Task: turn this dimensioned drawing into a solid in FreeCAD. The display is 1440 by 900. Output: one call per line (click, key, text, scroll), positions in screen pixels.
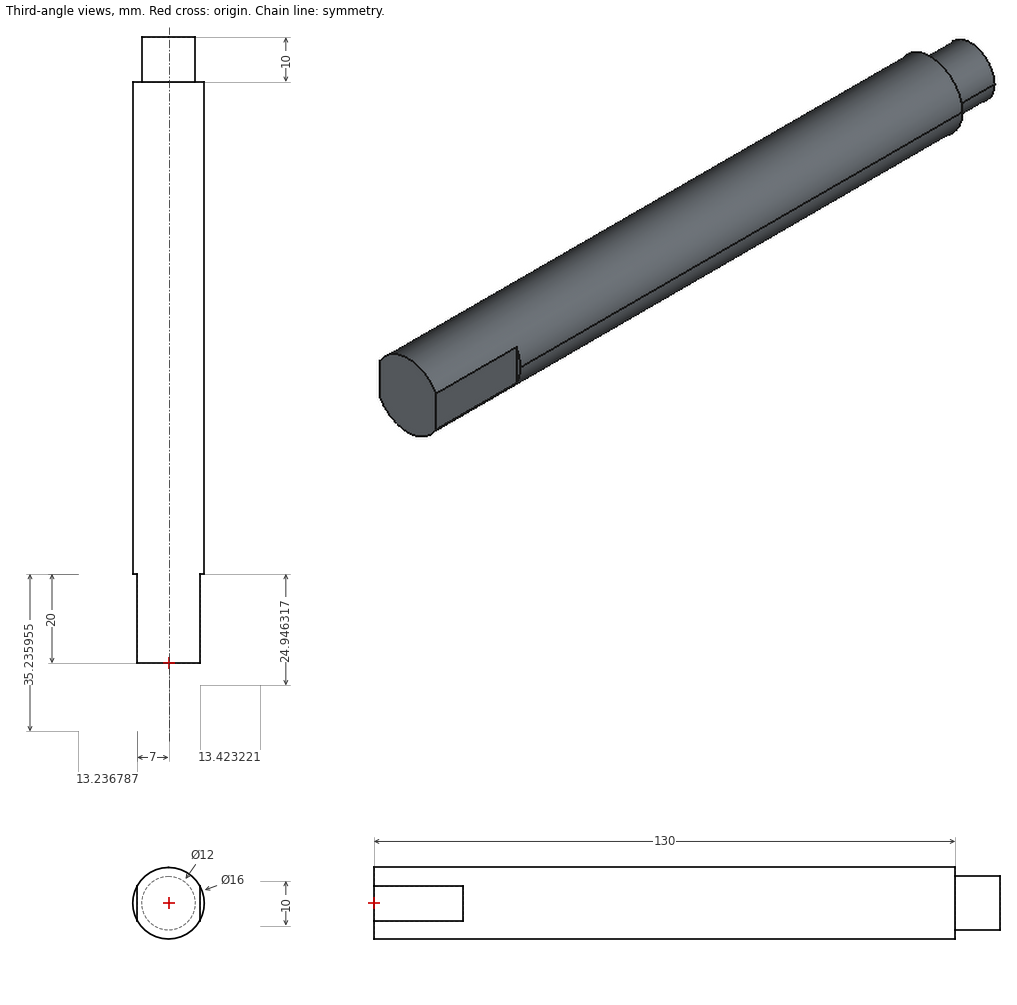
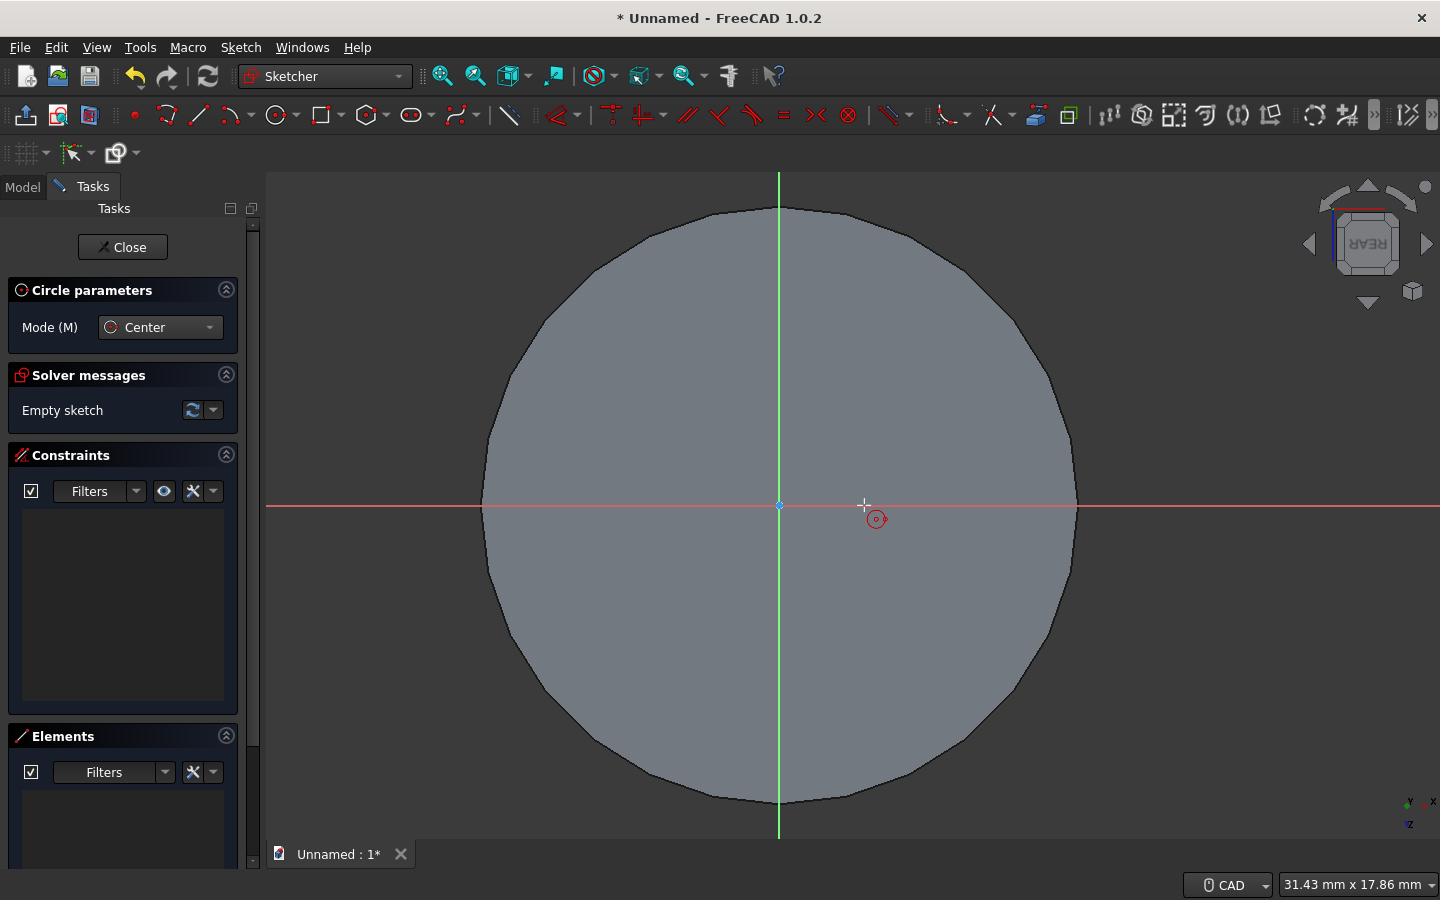
click(779, 505)
click(938, 347)
key(Escape)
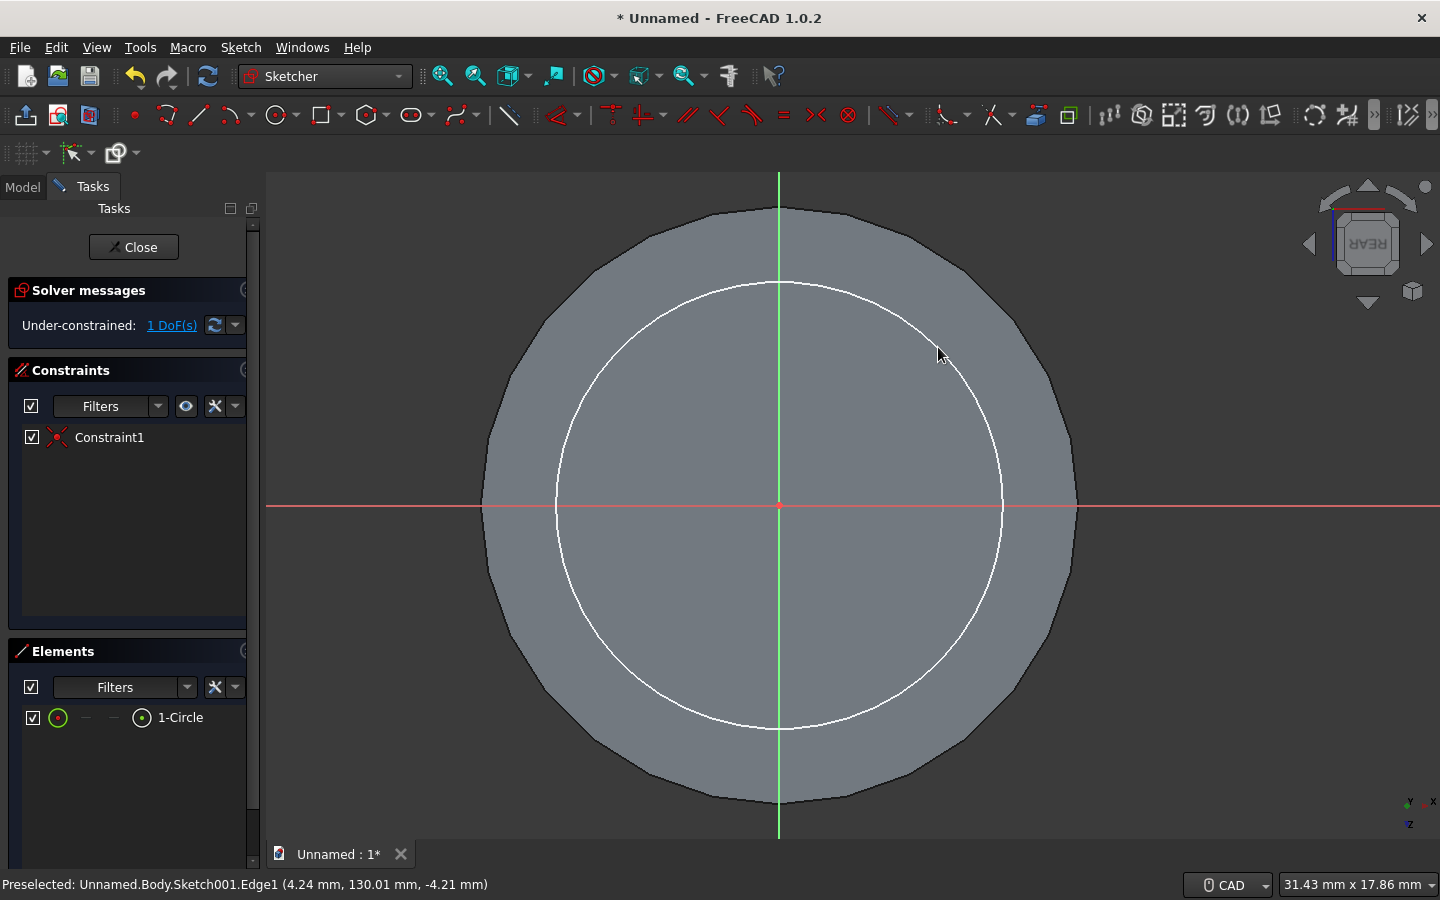
click(556, 116)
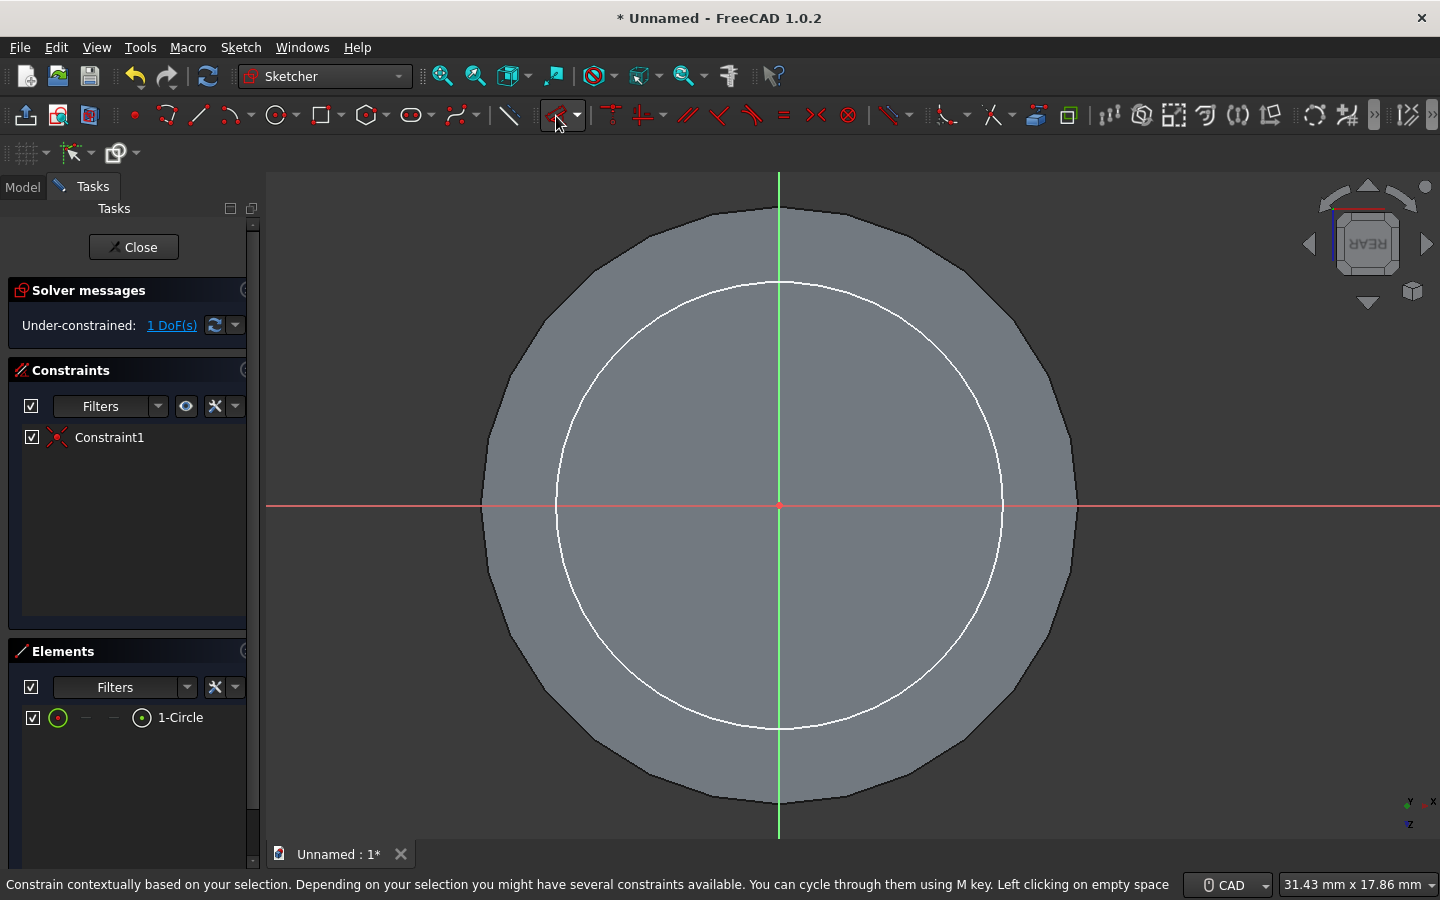
click(937, 347)
click(960, 324)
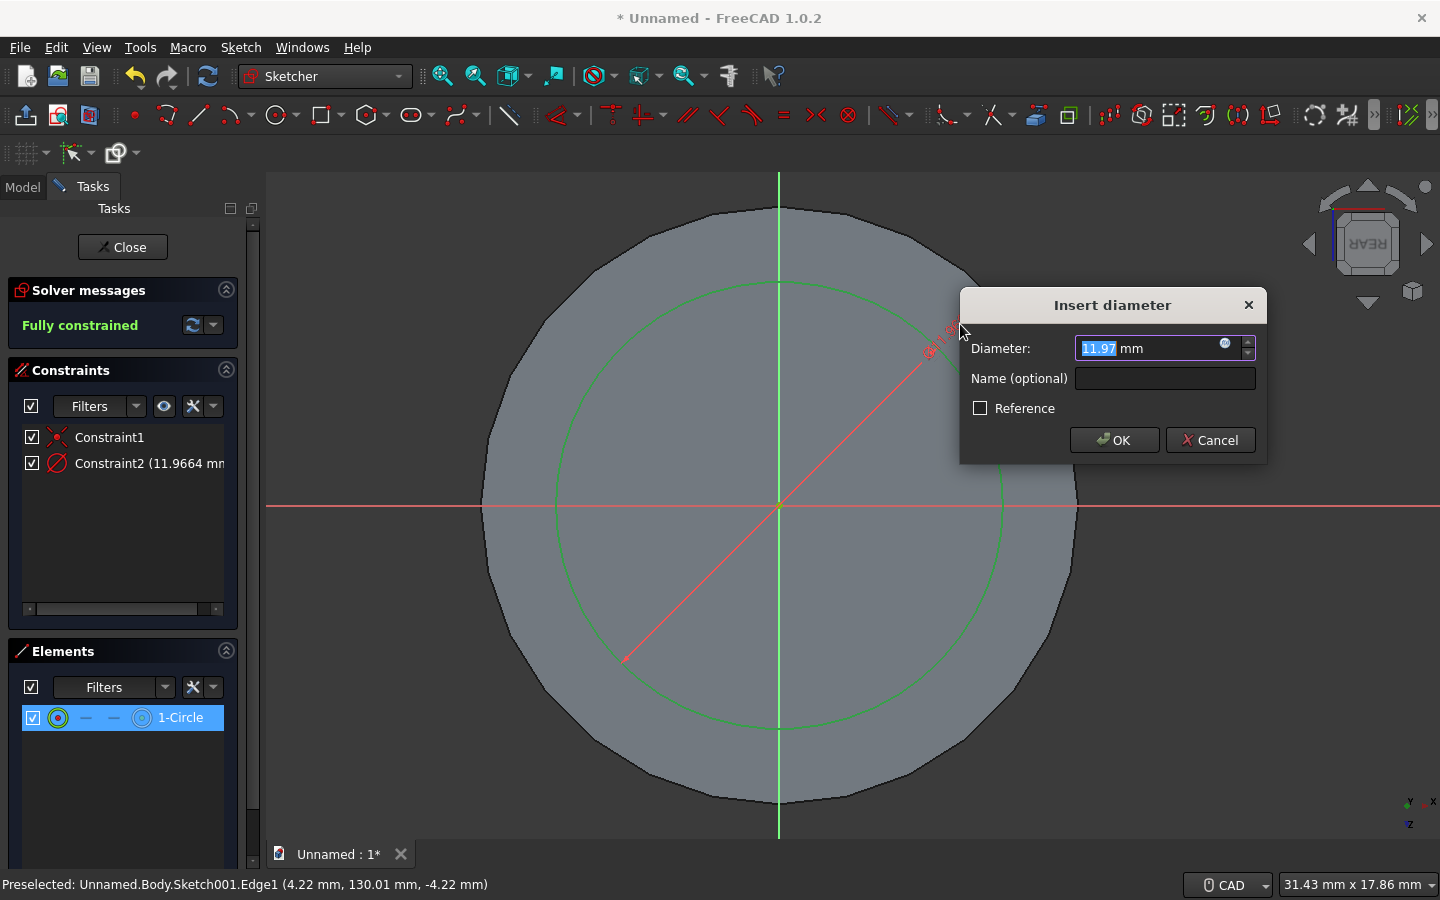
text(12)
key(Return)
key(Escape)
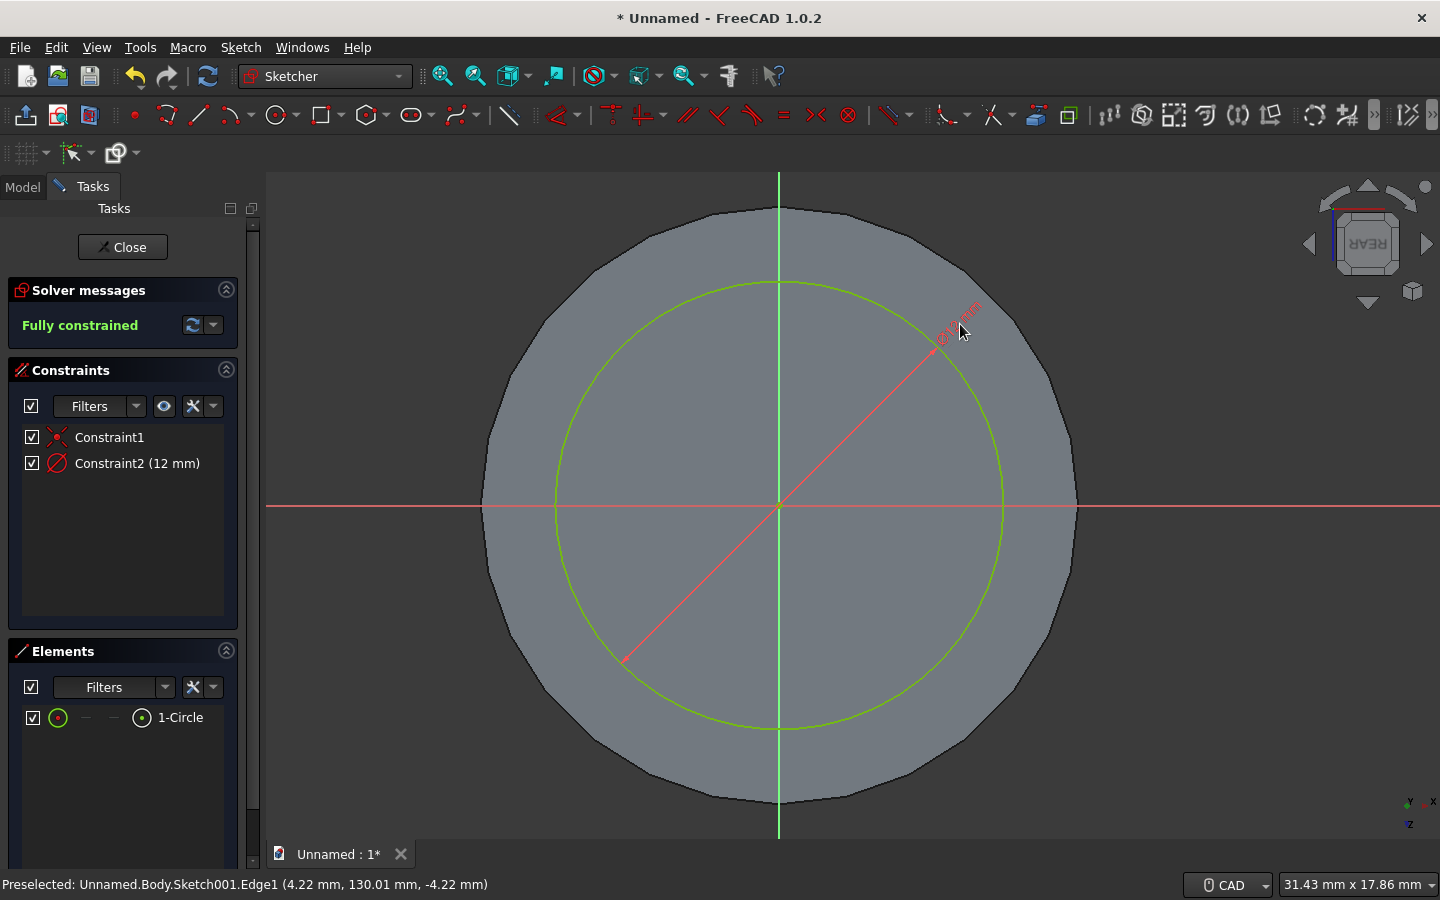
click(123, 247)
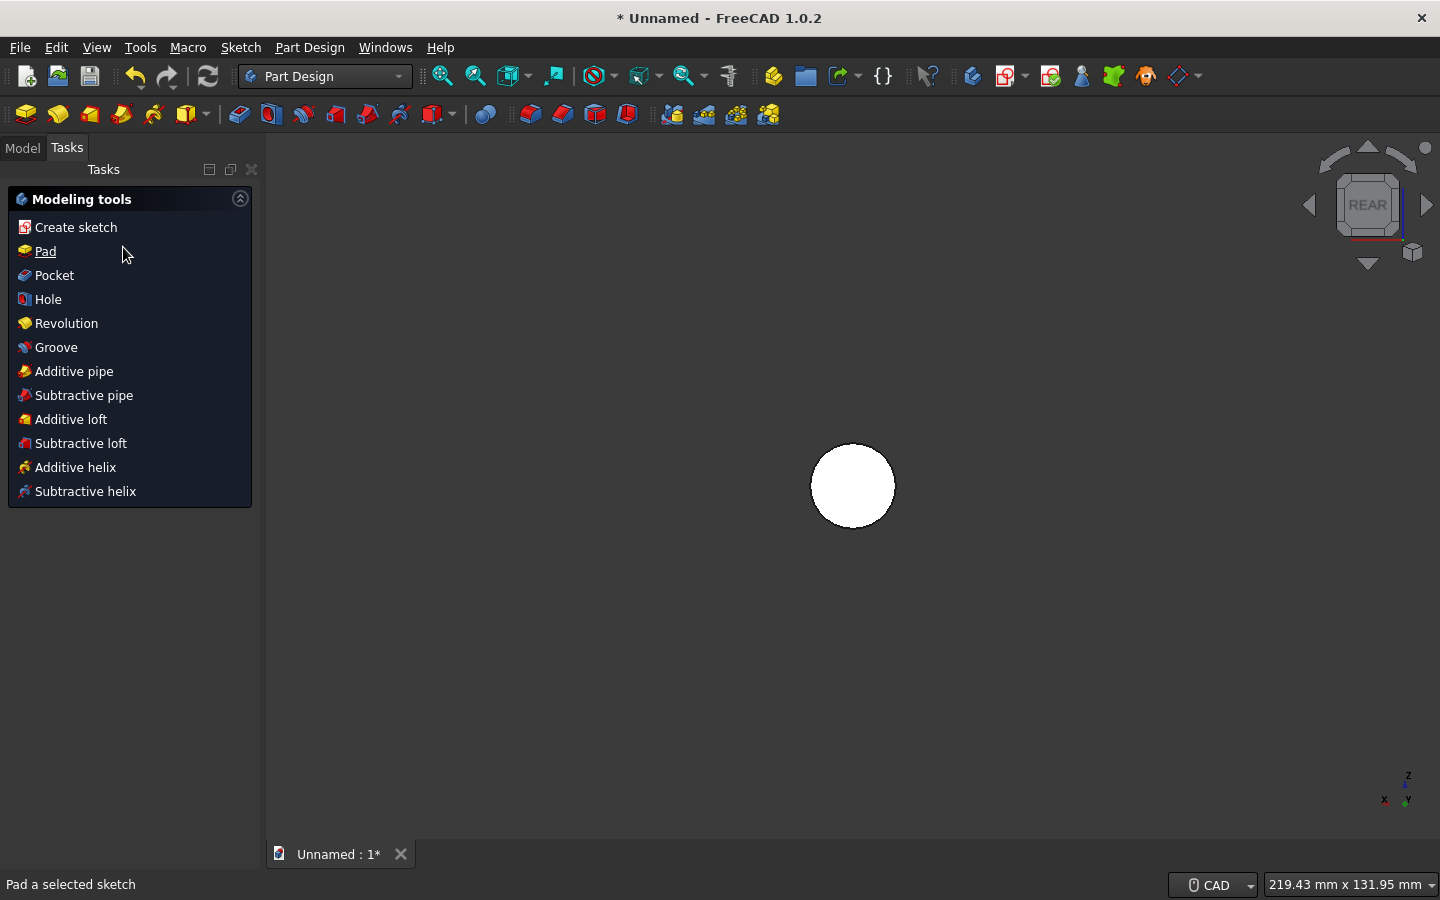
click(26, 114)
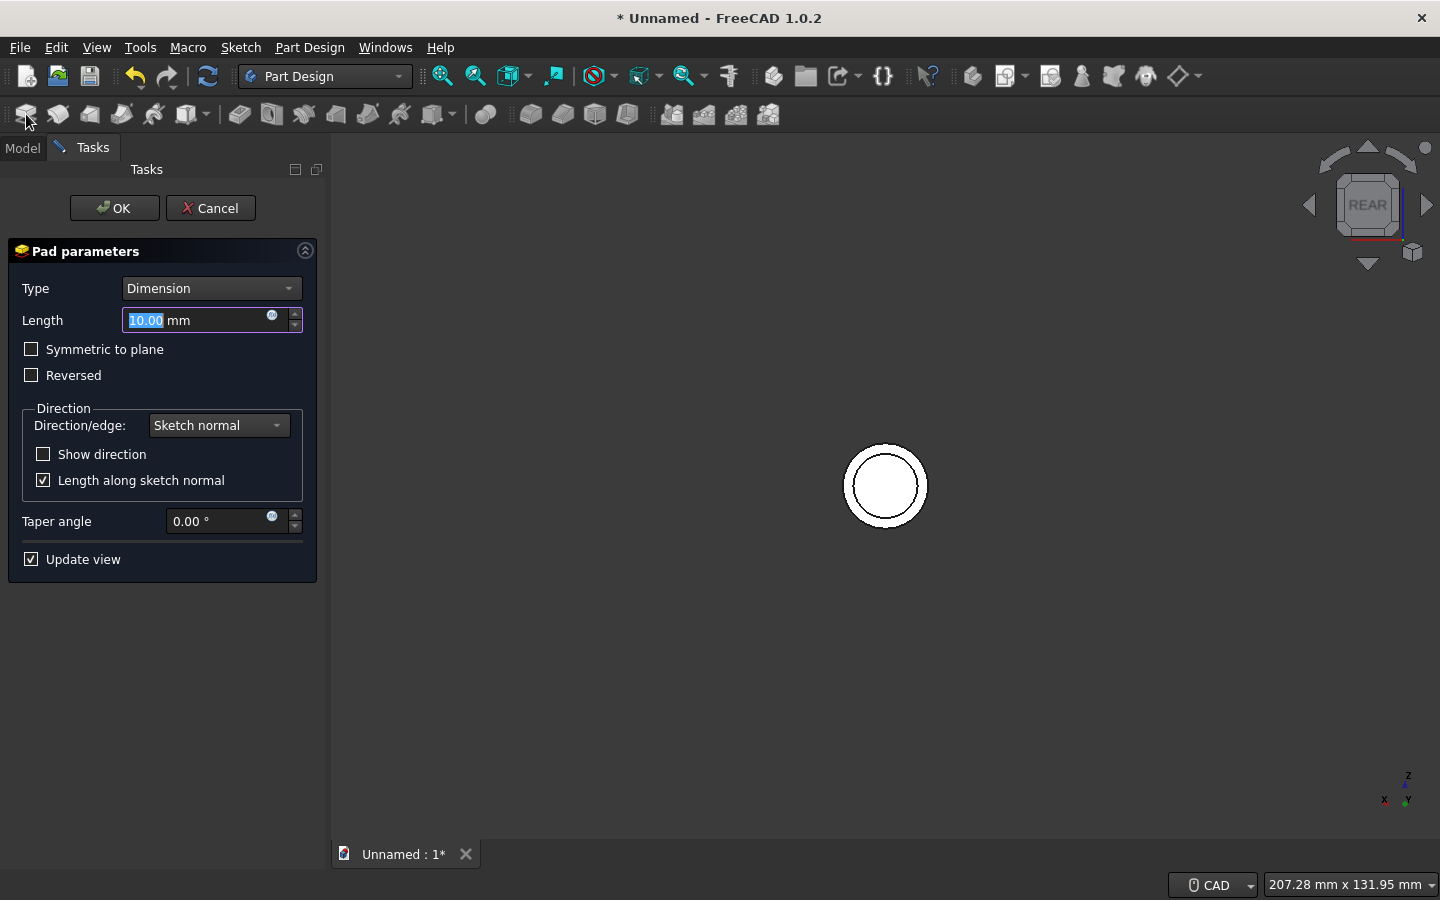
text(10)
key(Tab)